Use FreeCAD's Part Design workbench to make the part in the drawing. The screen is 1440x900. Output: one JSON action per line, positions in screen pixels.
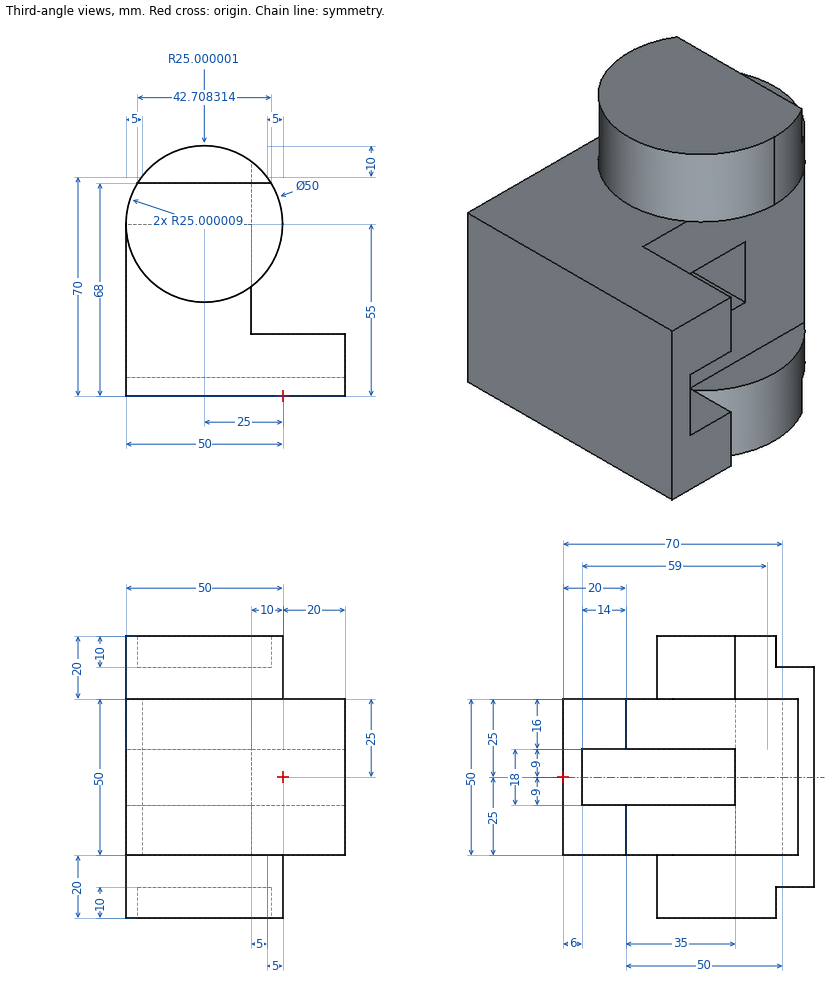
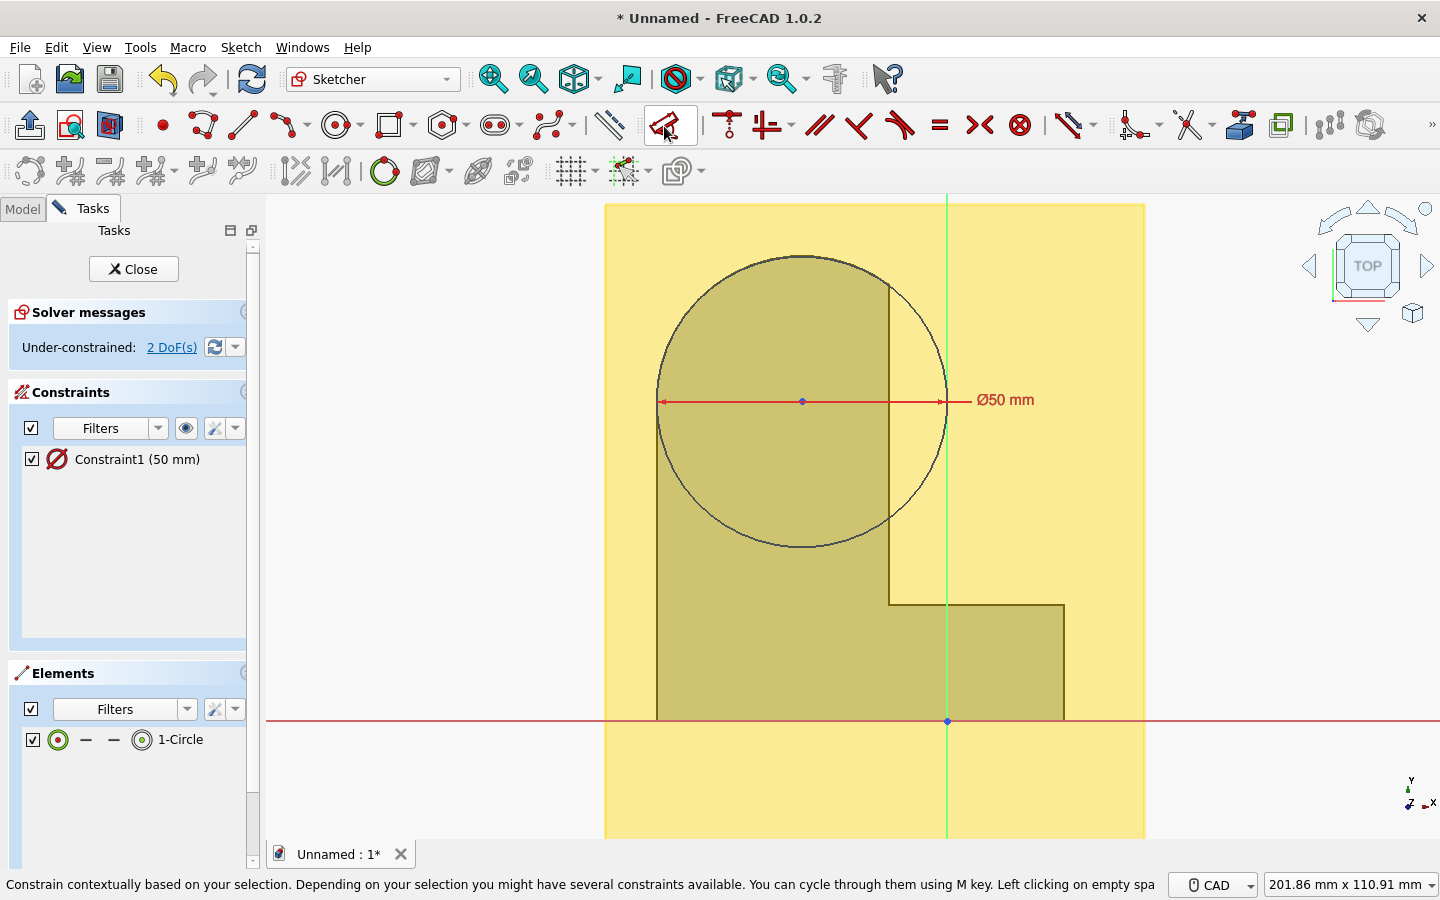
{"action": "left_click", "coordinate": [802, 402]}
{"action": "left_click", "coordinate": [875, 755]}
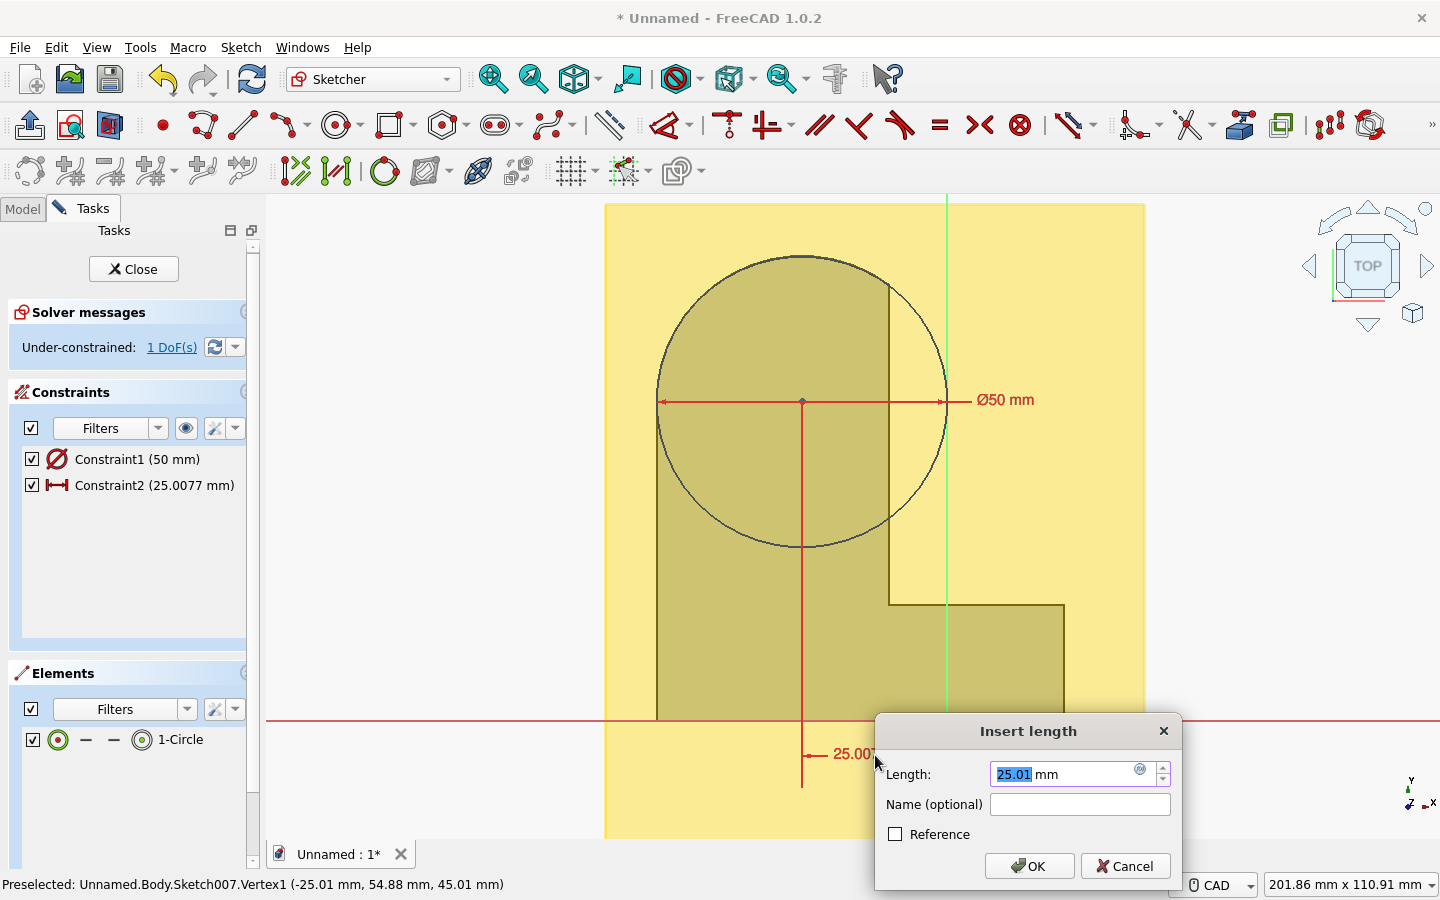
{"action": "type", "text": "25"}
{"action": "key", "text": "Return"}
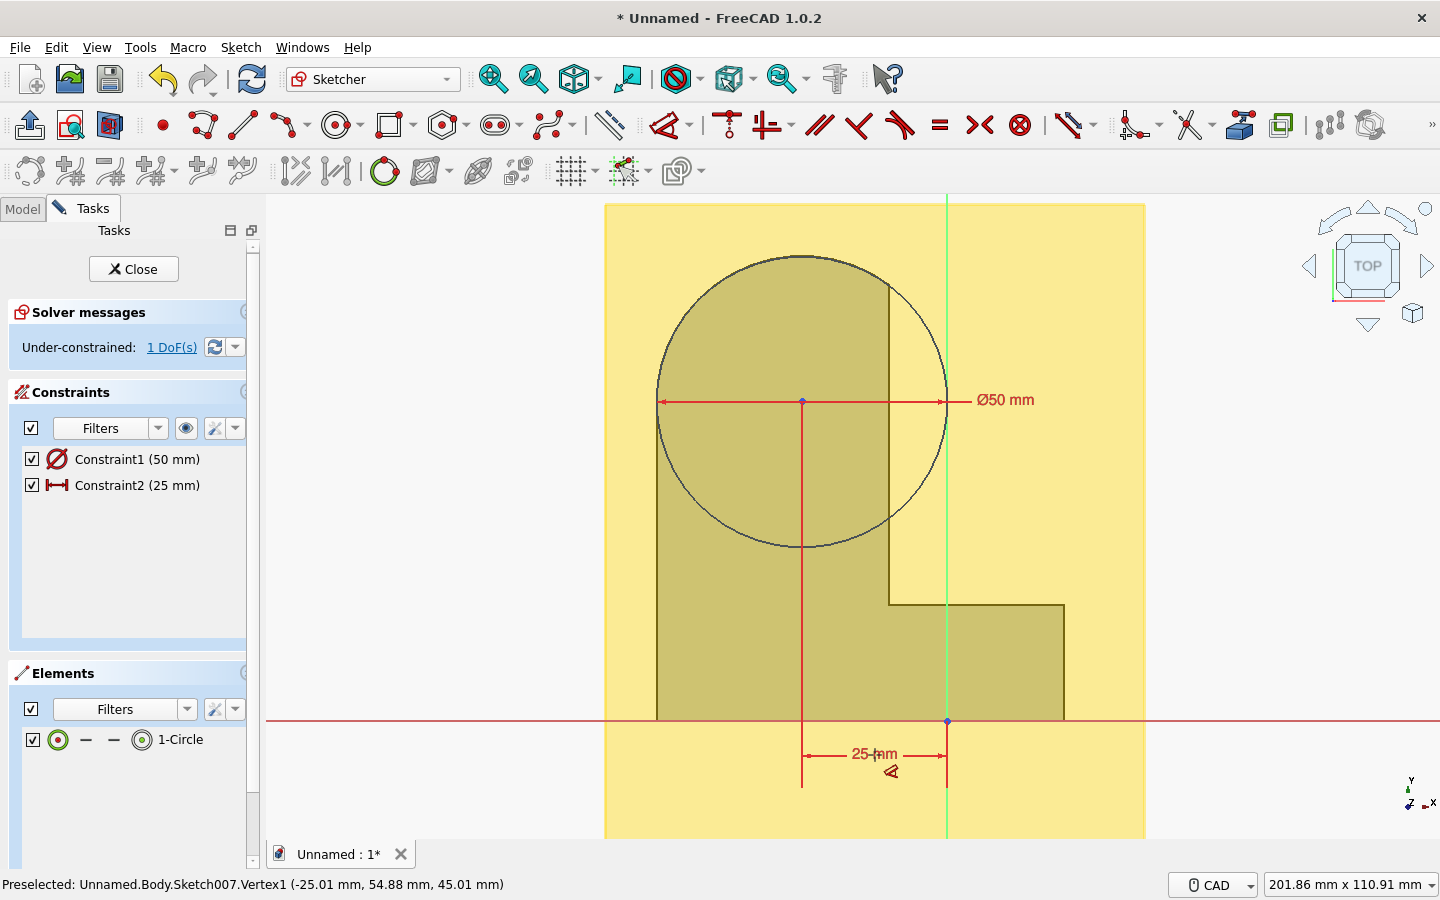
{"action": "left_click", "coordinate": [802, 402]}
{"action": "left_click", "coordinate": [981, 562]}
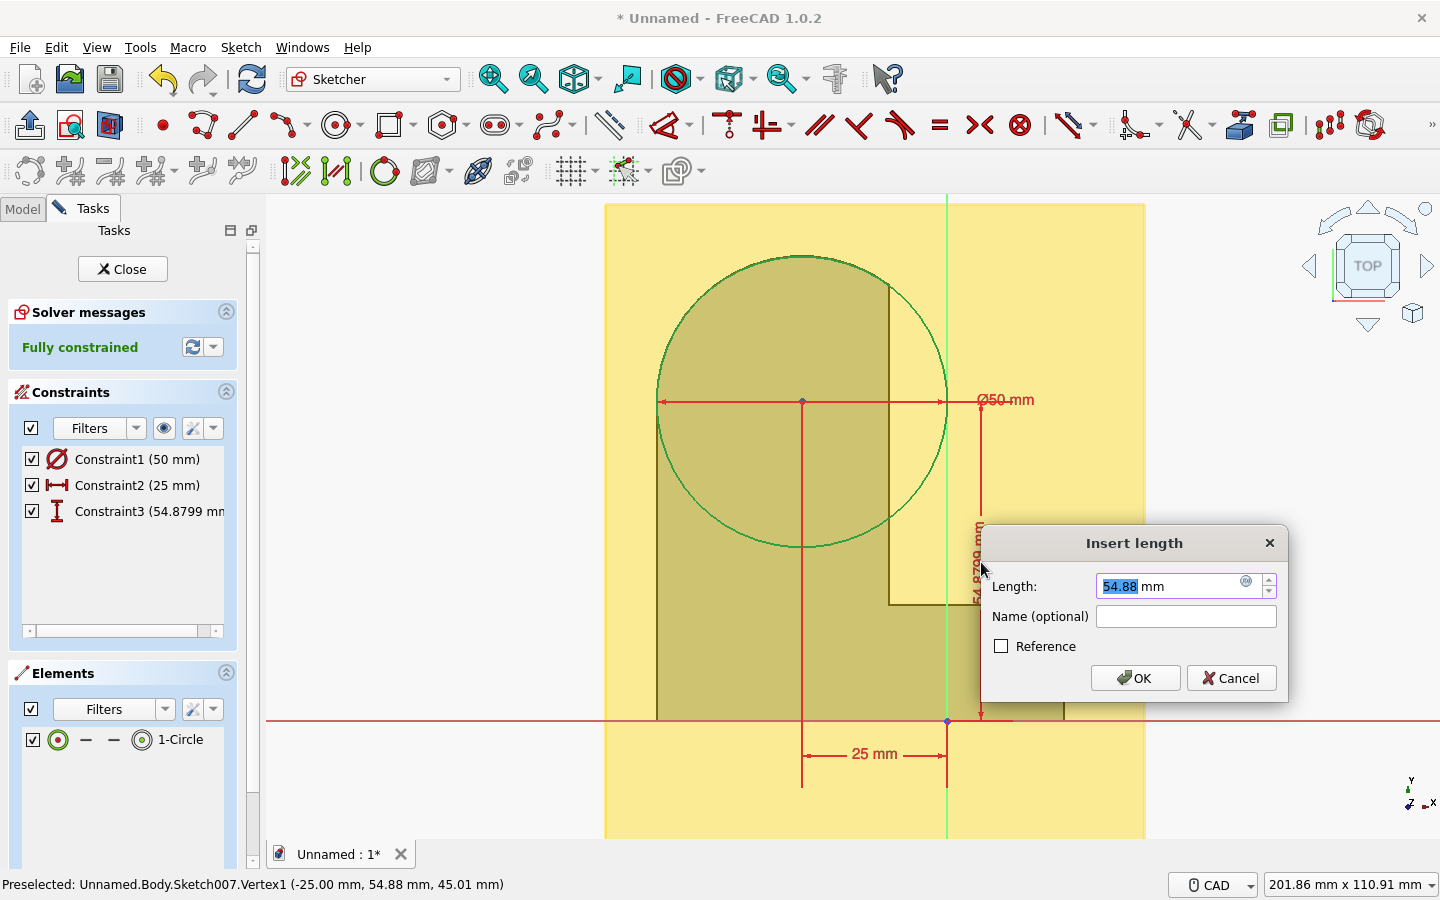
{"action": "type", "text": "55"}
{"action": "key", "text": "Return"}
{"action": "key", "text": "Escape"}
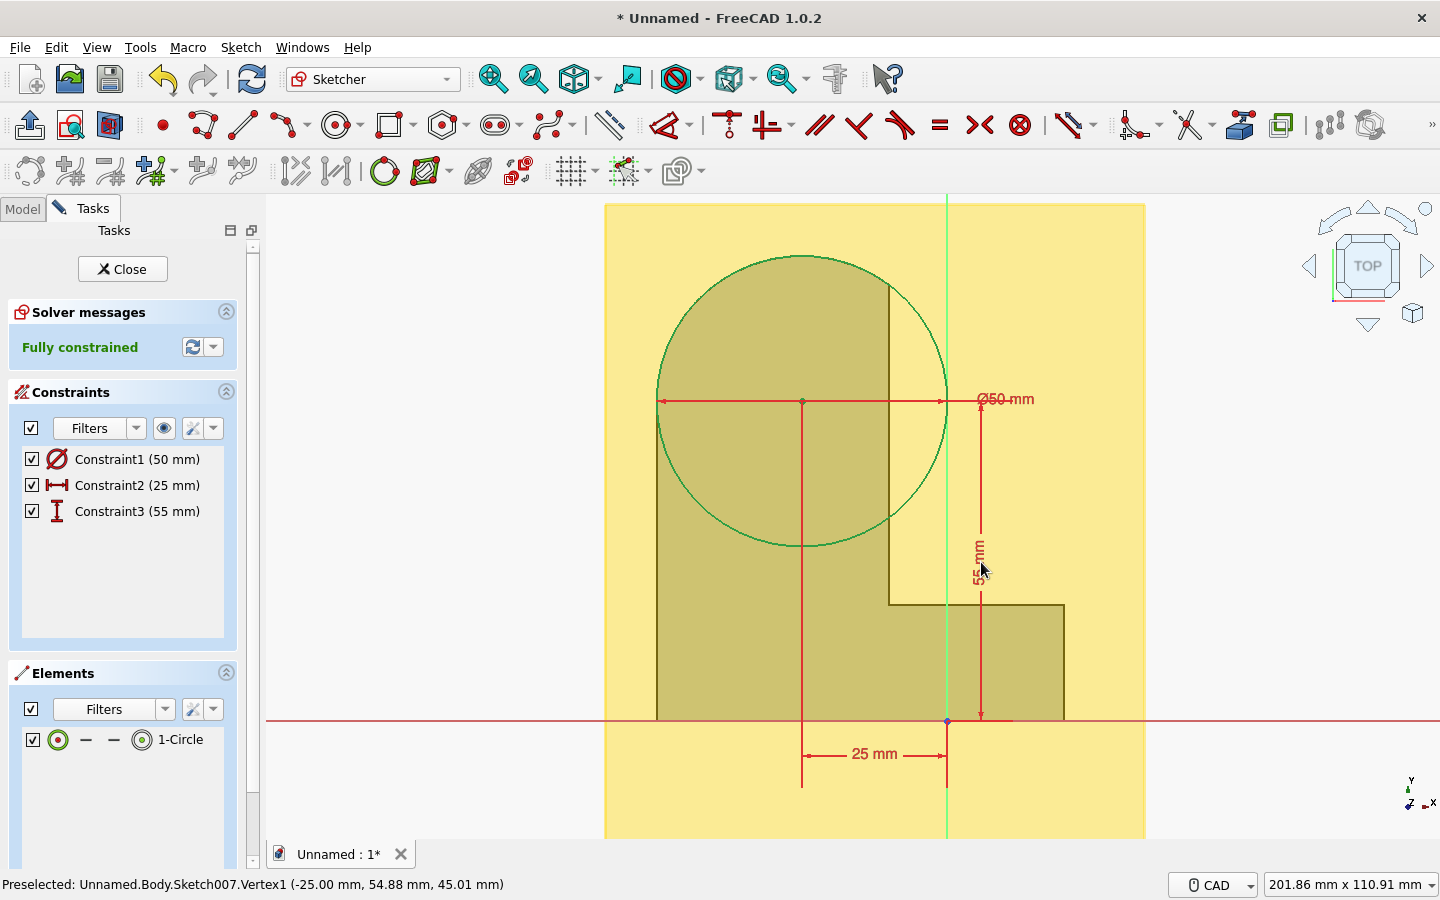
{"action": "left_click", "coordinate": [123, 269]}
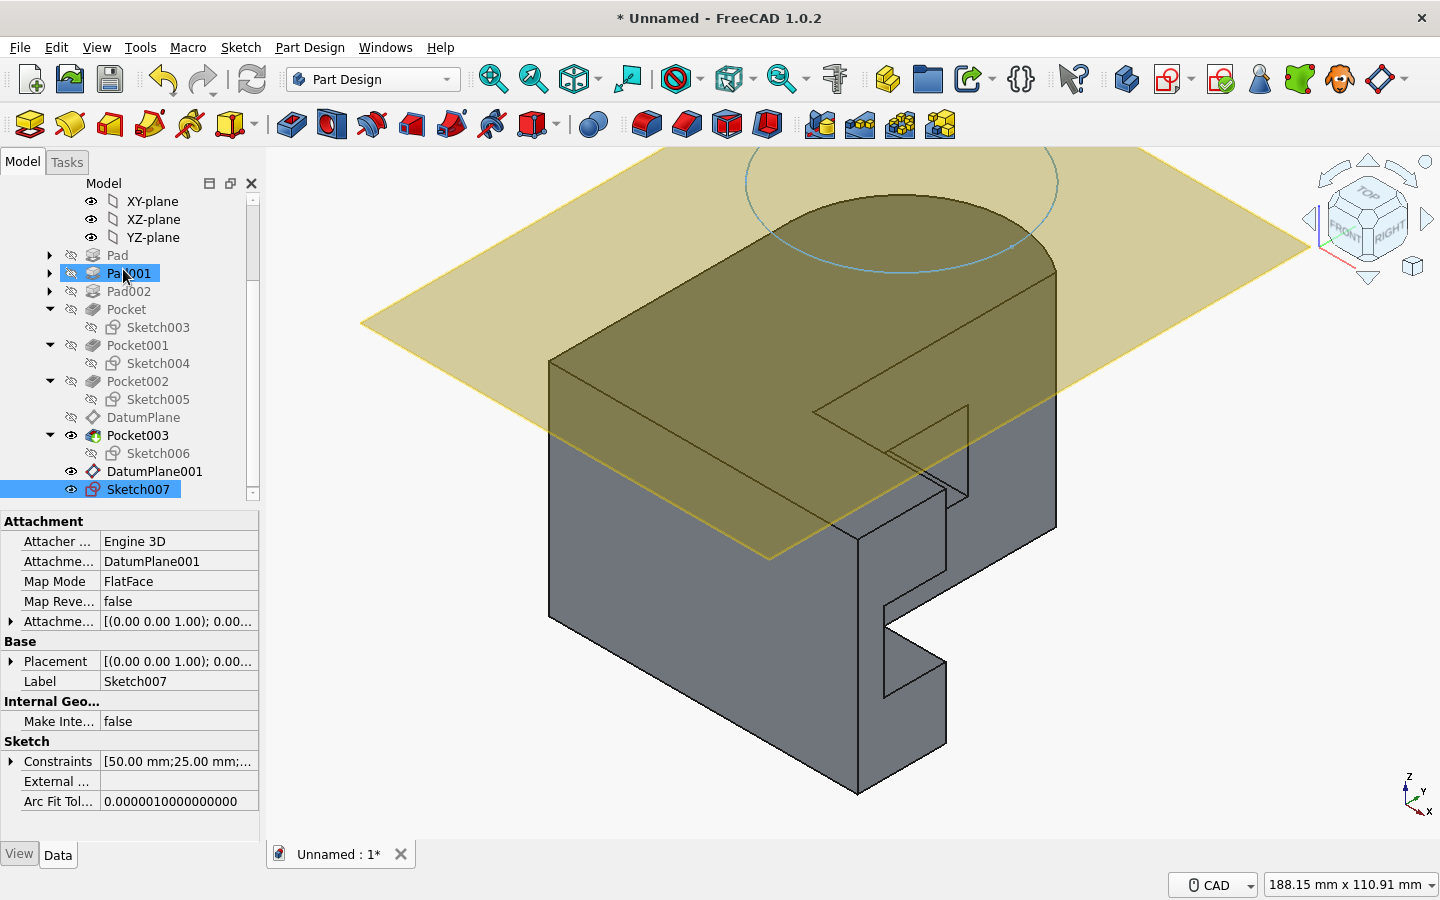
{"action": "left_click", "coordinate": [30, 124]}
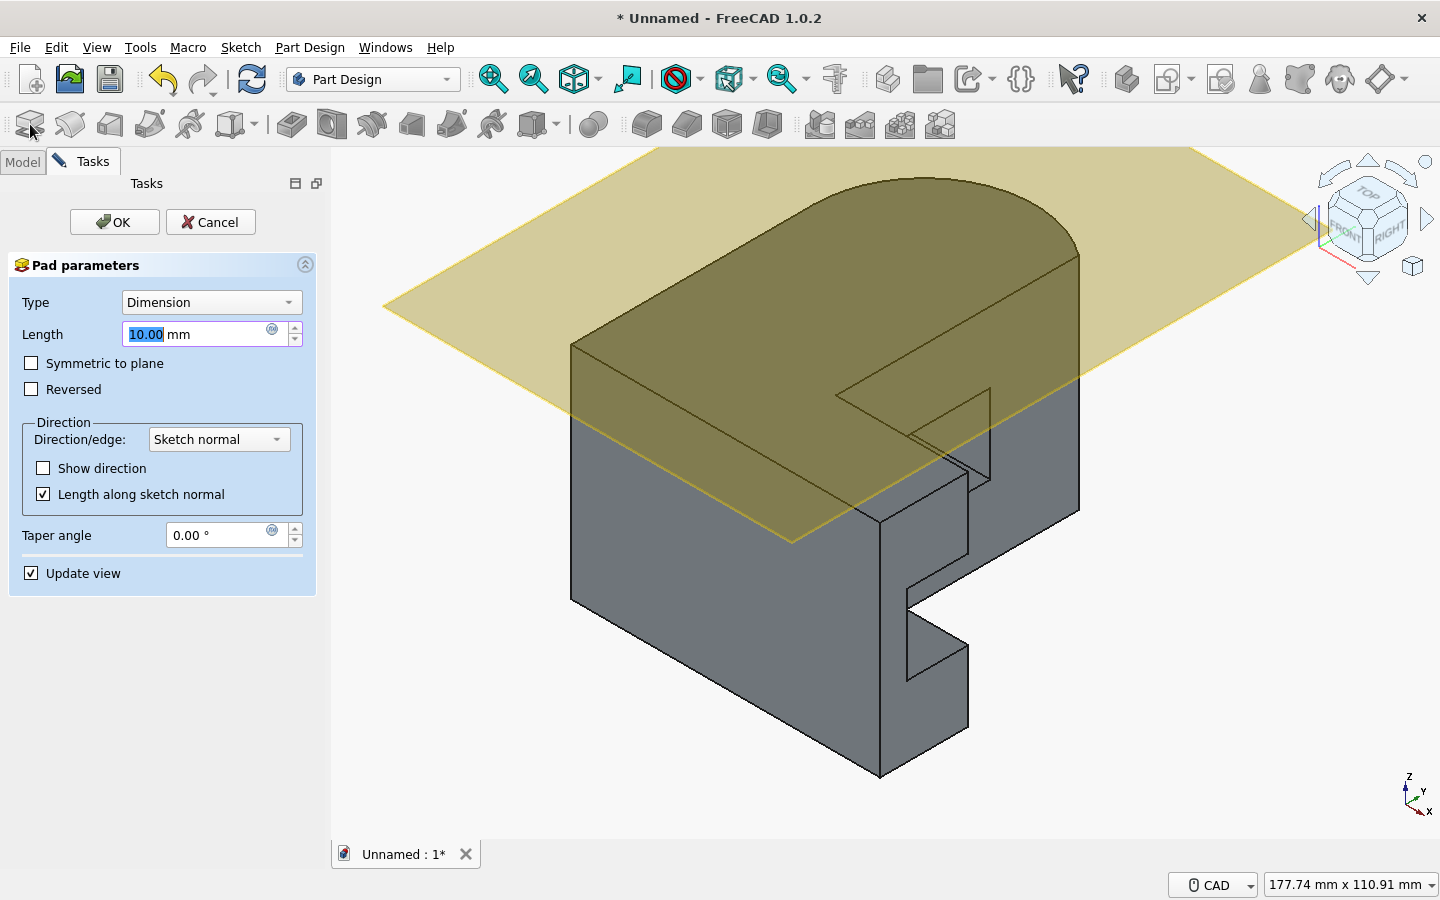
{"action": "type", "text": "20"}
{"action": "key", "text": "Tab"}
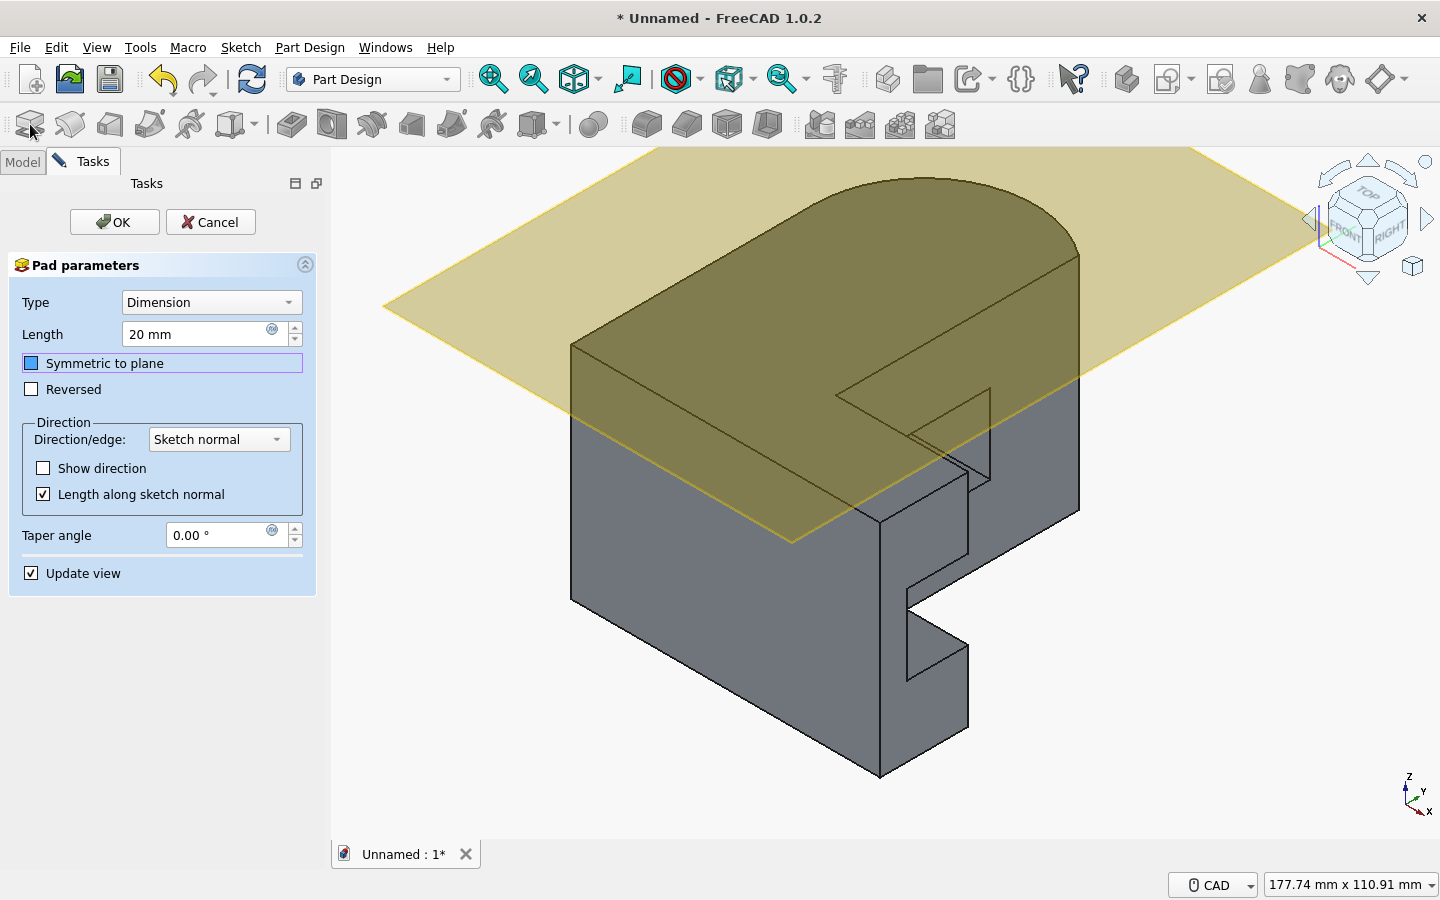
{"action": "left_click", "coordinate": [30, 389]}